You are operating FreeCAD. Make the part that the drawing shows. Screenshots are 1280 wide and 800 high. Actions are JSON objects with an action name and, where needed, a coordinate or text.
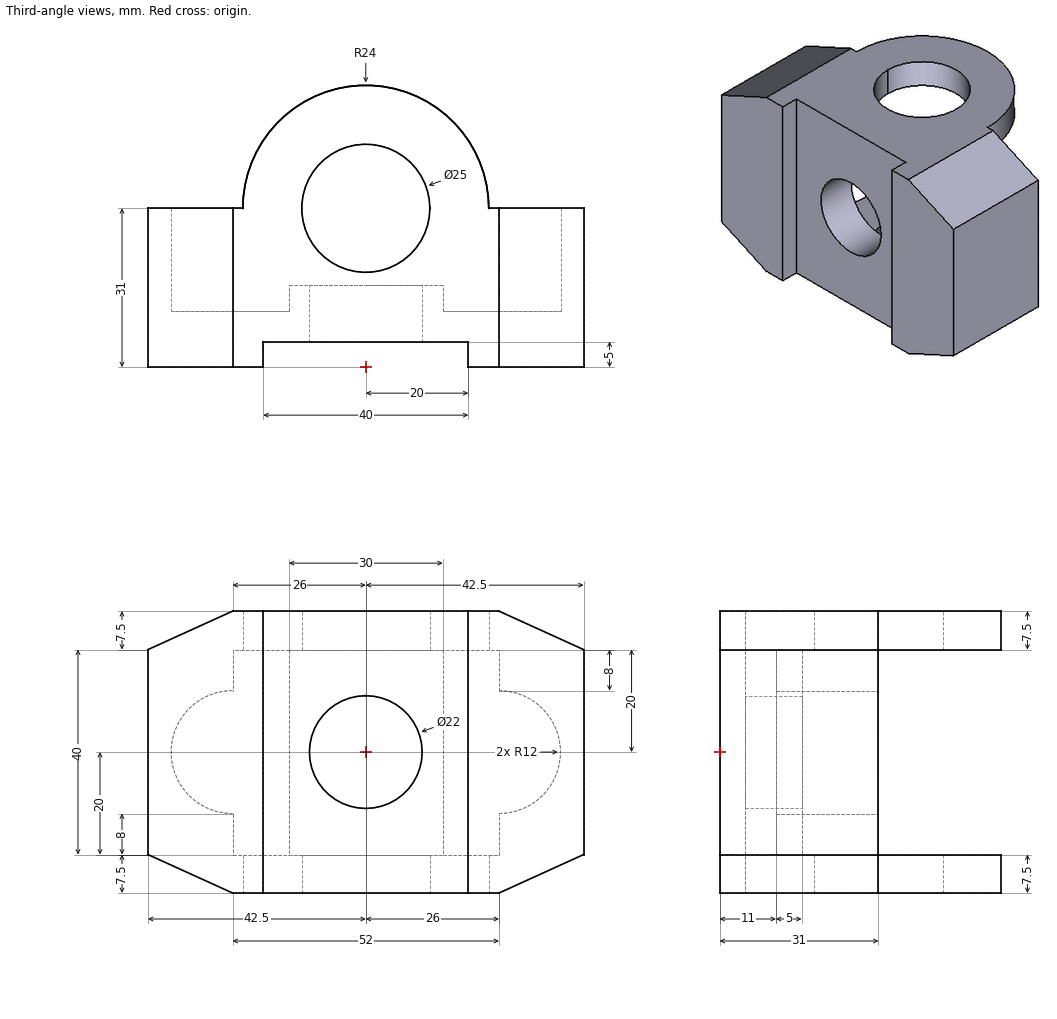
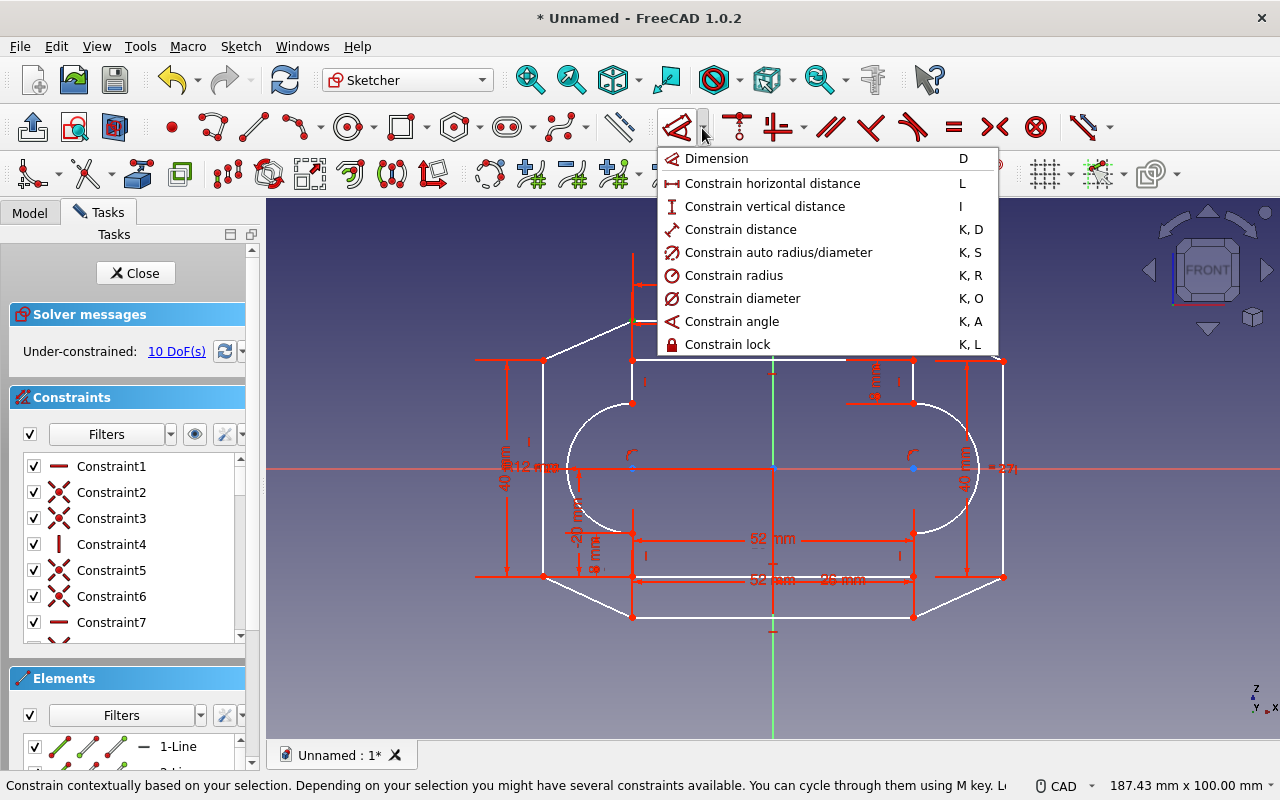
{"action": "left_click", "coordinate": [828, 184]}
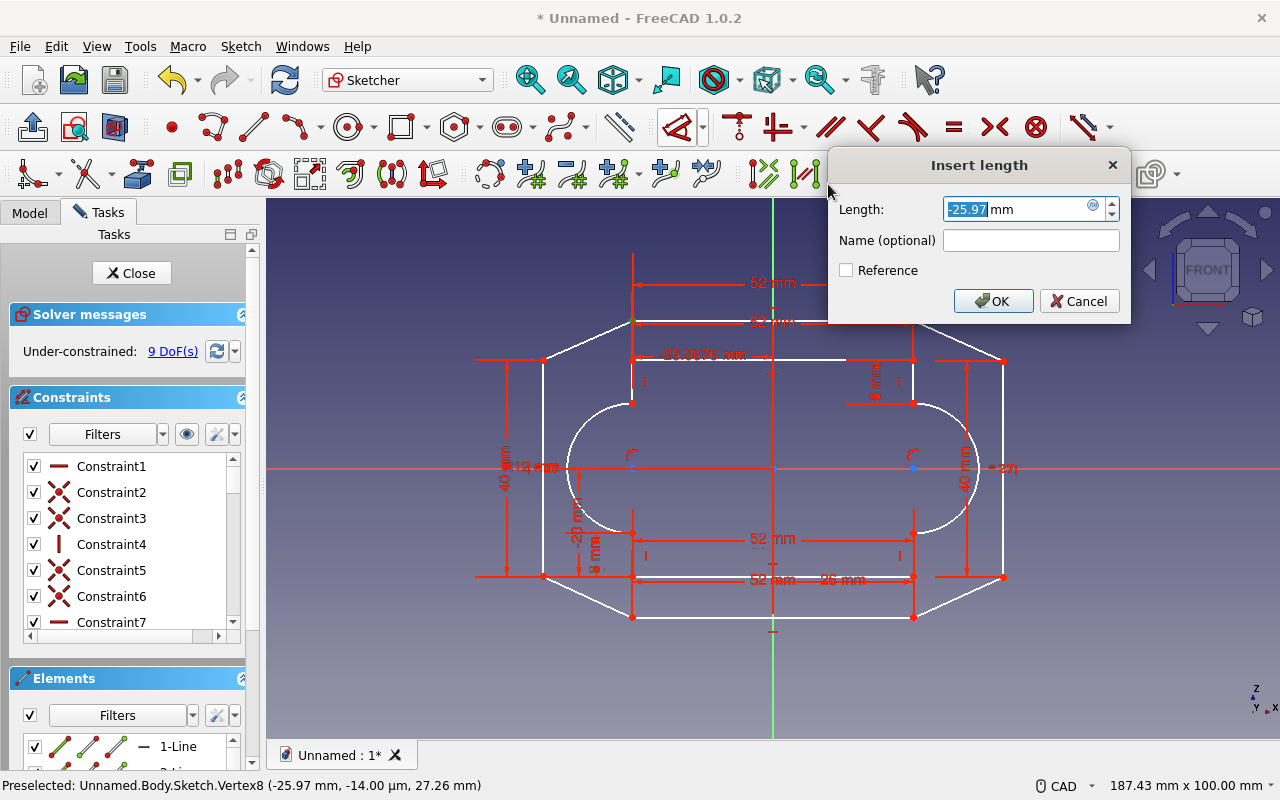
{"action": "type", "text": "-26"}
{"action": "key", "text": "Return"}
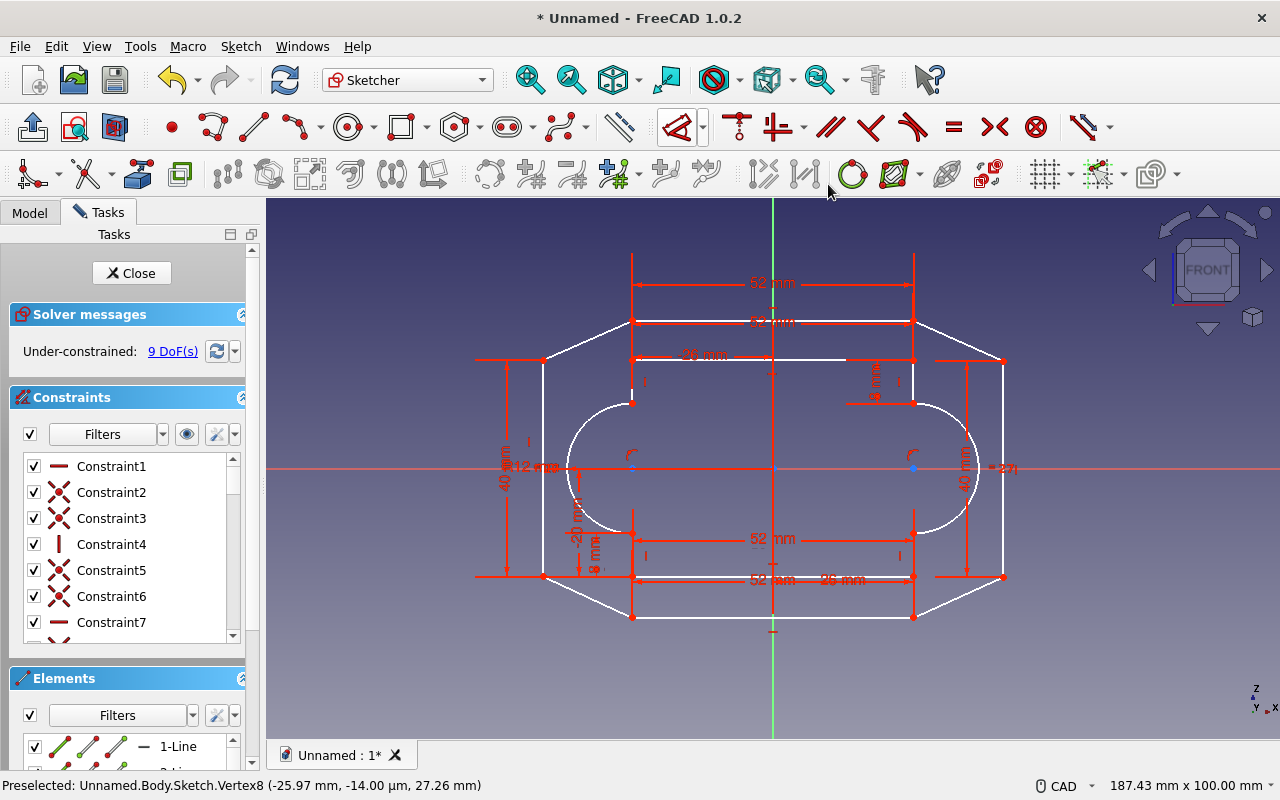
{"action": "left_click", "coordinate": [1003, 361]}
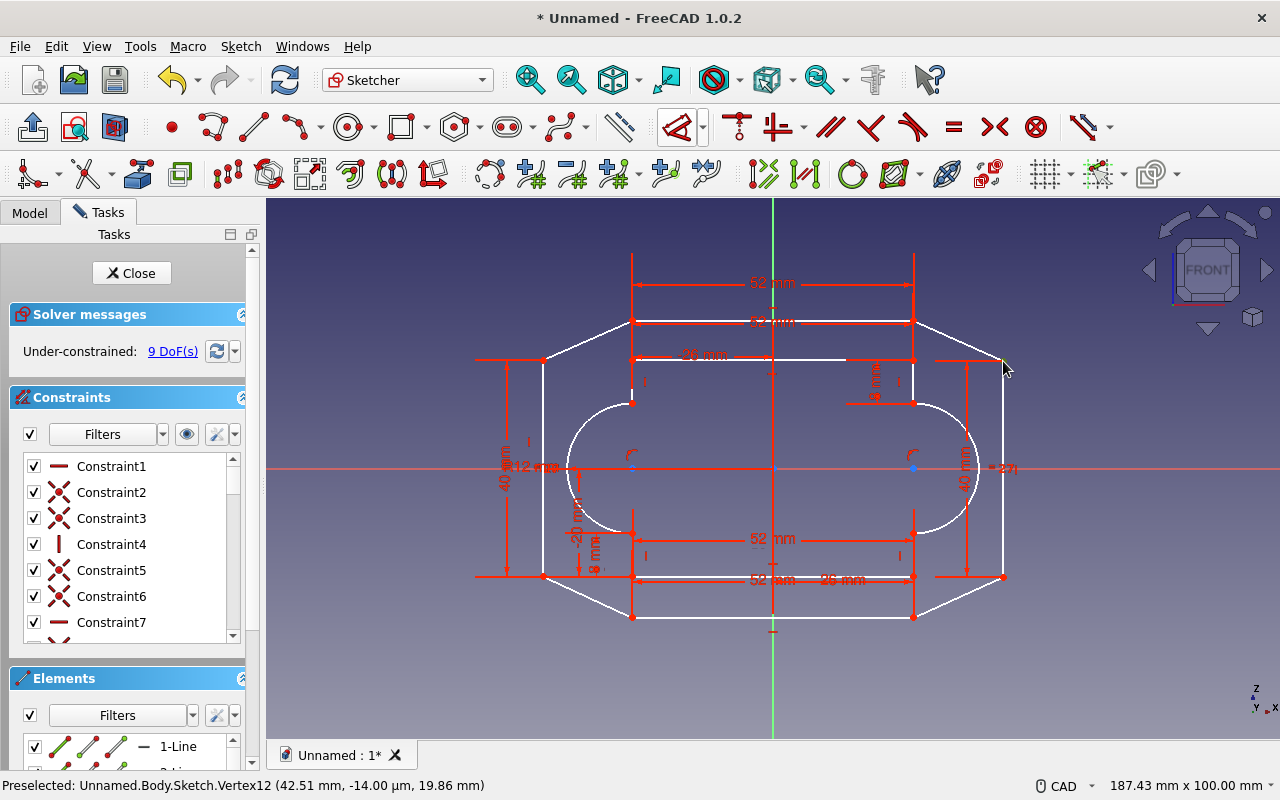
{"action": "left_click", "coordinate": [702, 128]}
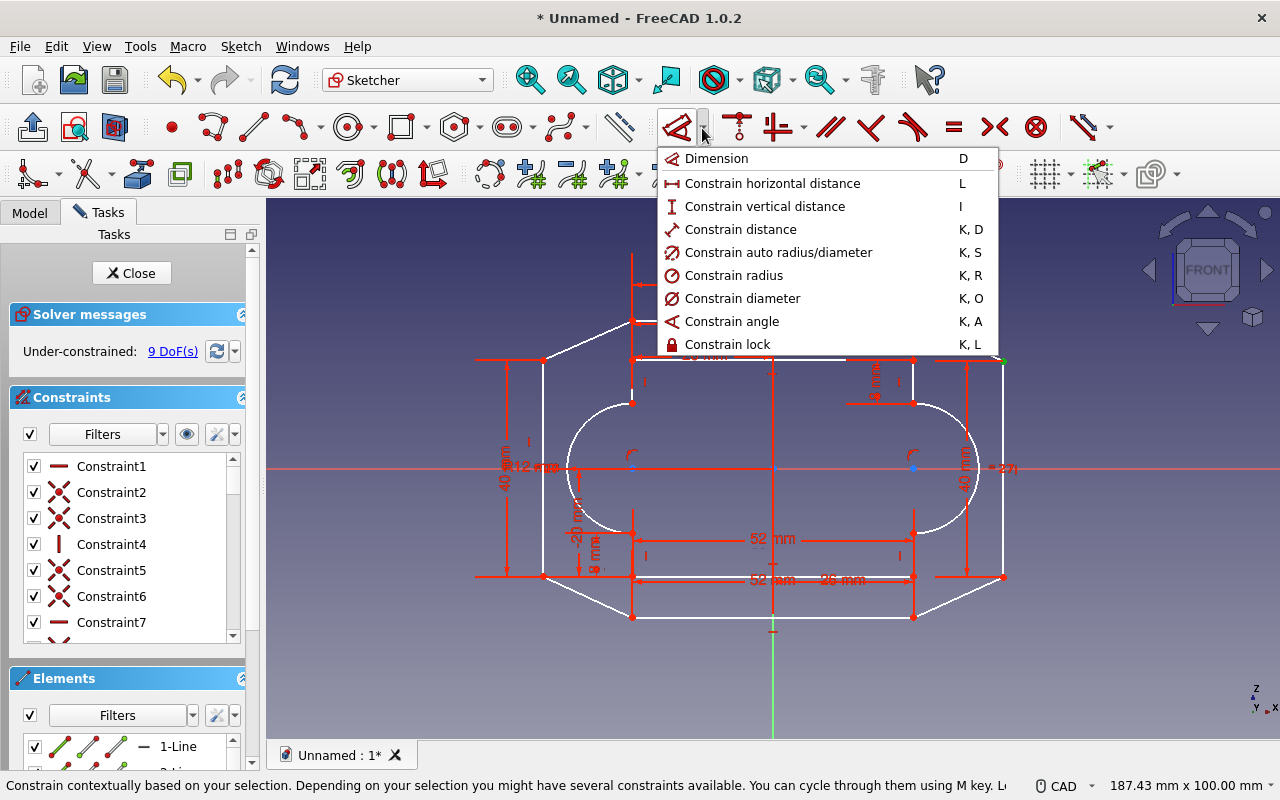
{"action": "left_click", "coordinate": [828, 206]}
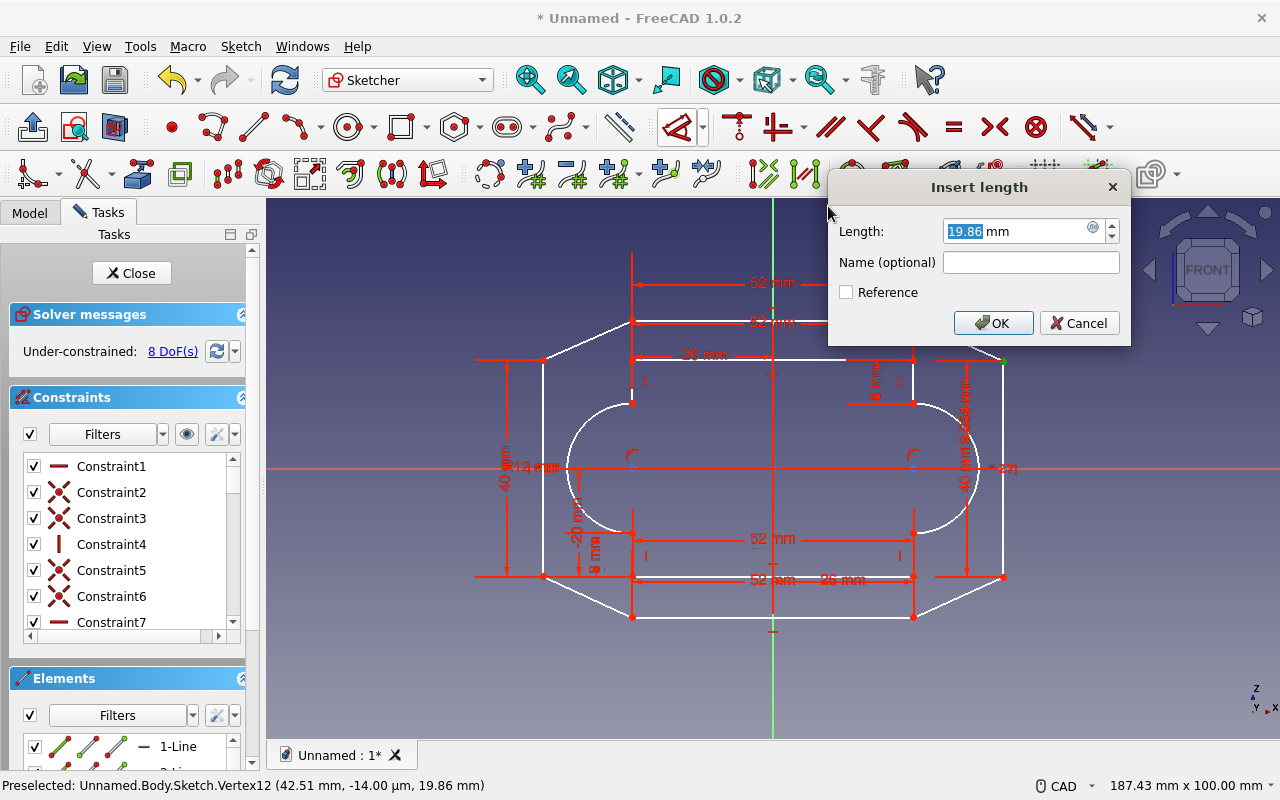
{"action": "type", "text": "20"}
{"action": "key", "text": "Return"}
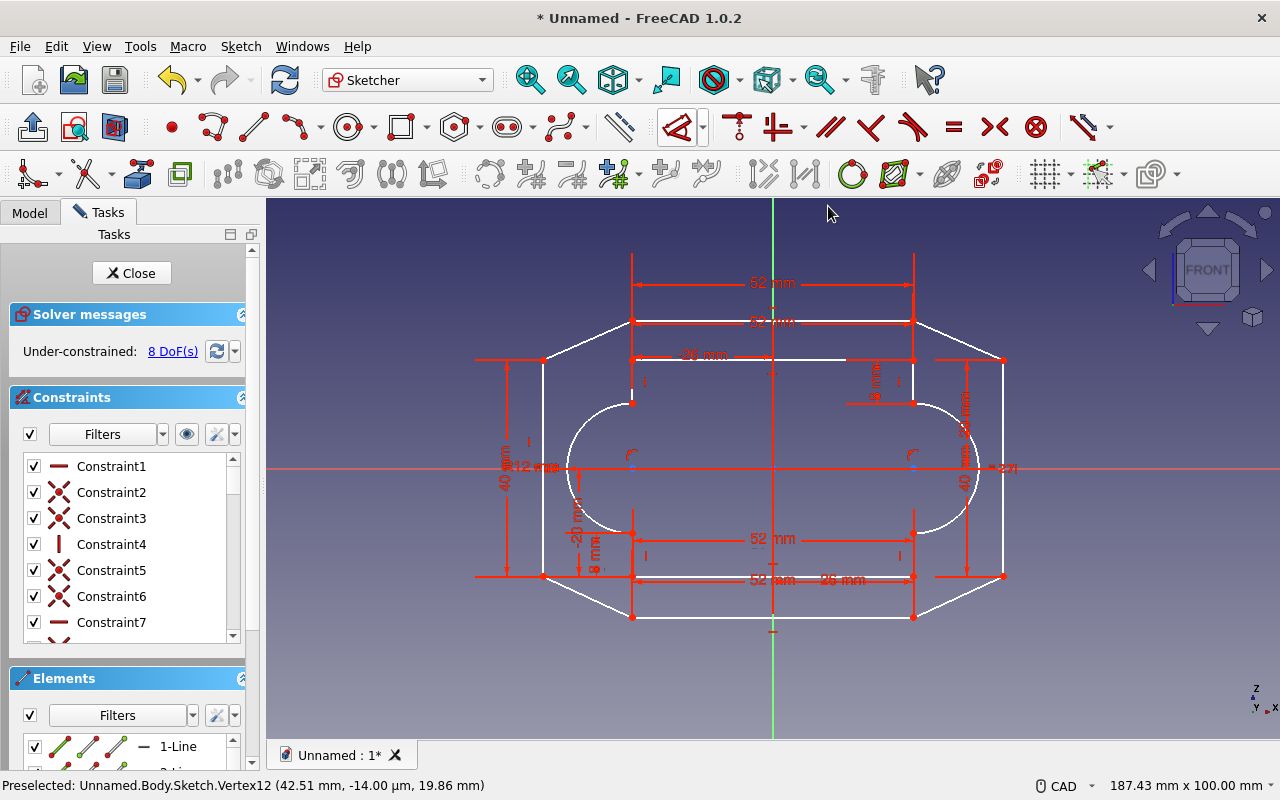
{"action": "left_click", "coordinate": [913, 404]}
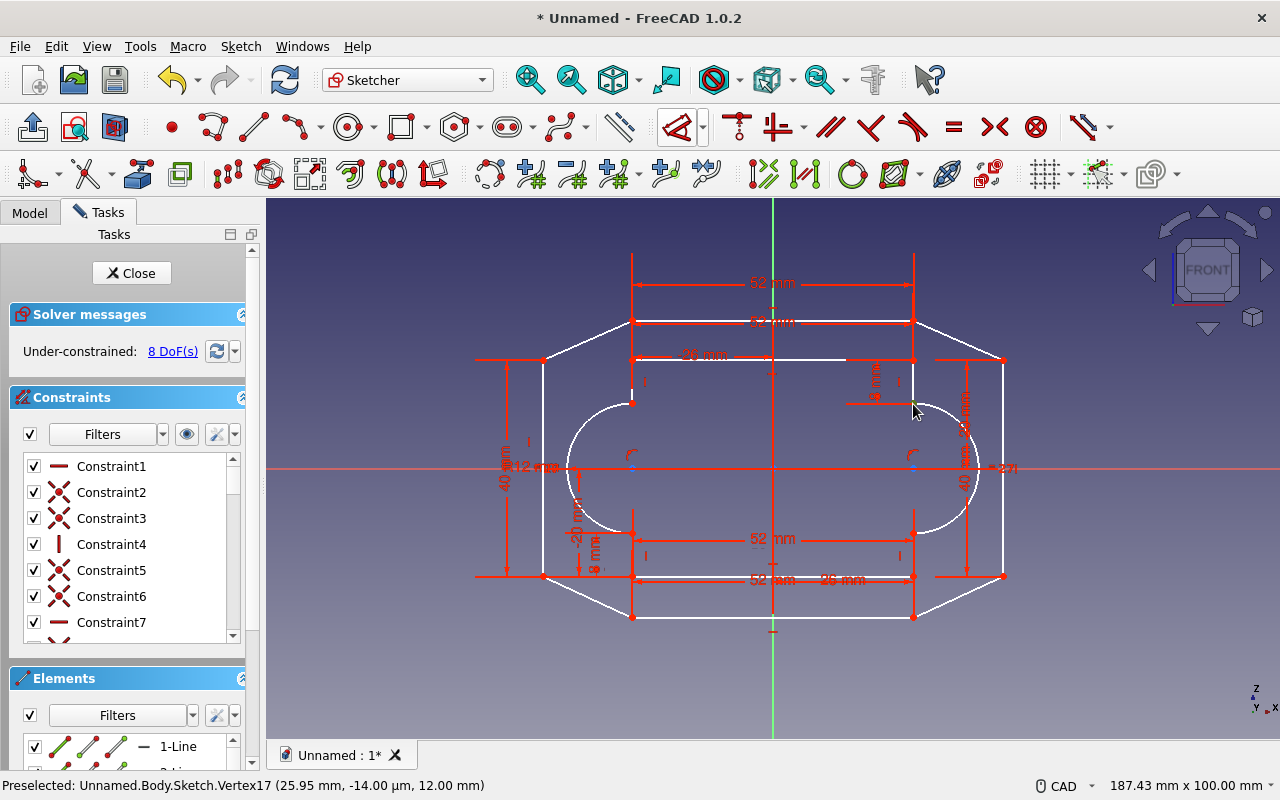
{"action": "key", "text": "l"}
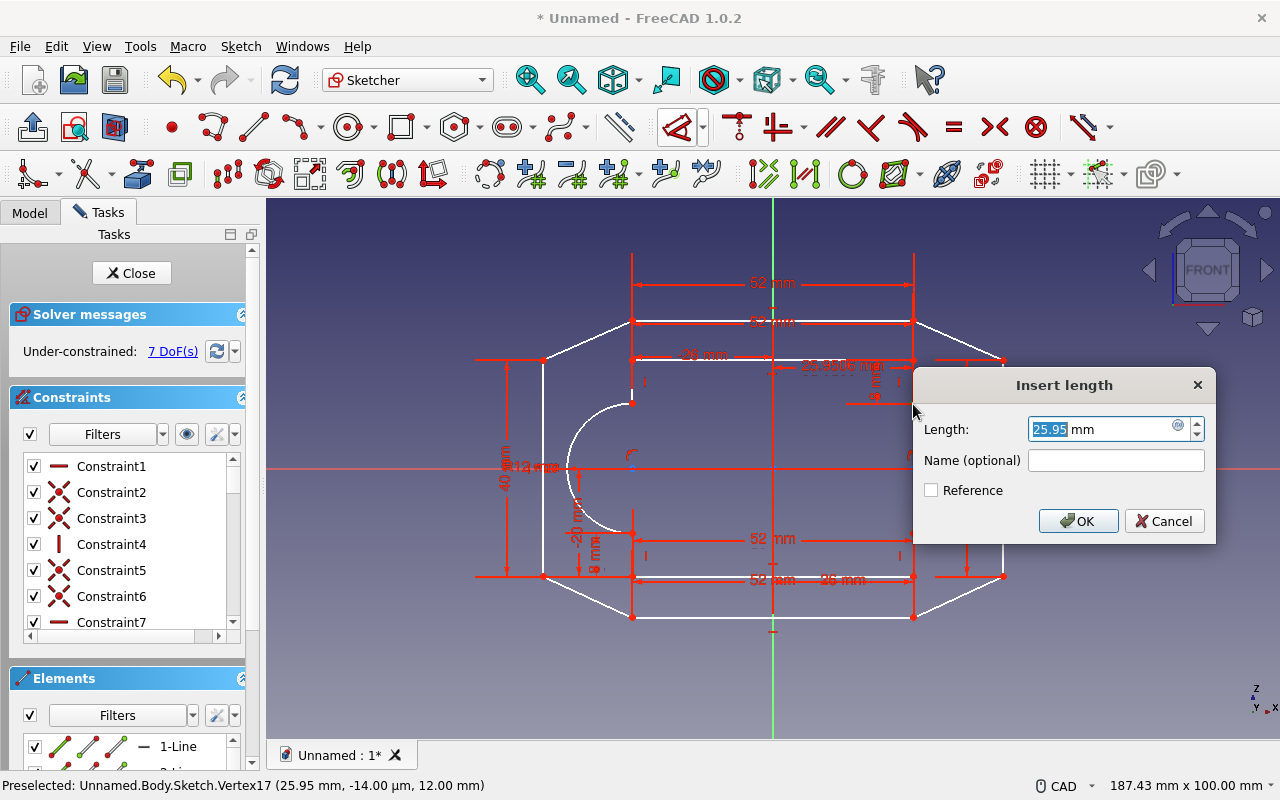
{"action": "type", "text": "26"}
{"action": "key", "text": "Return"}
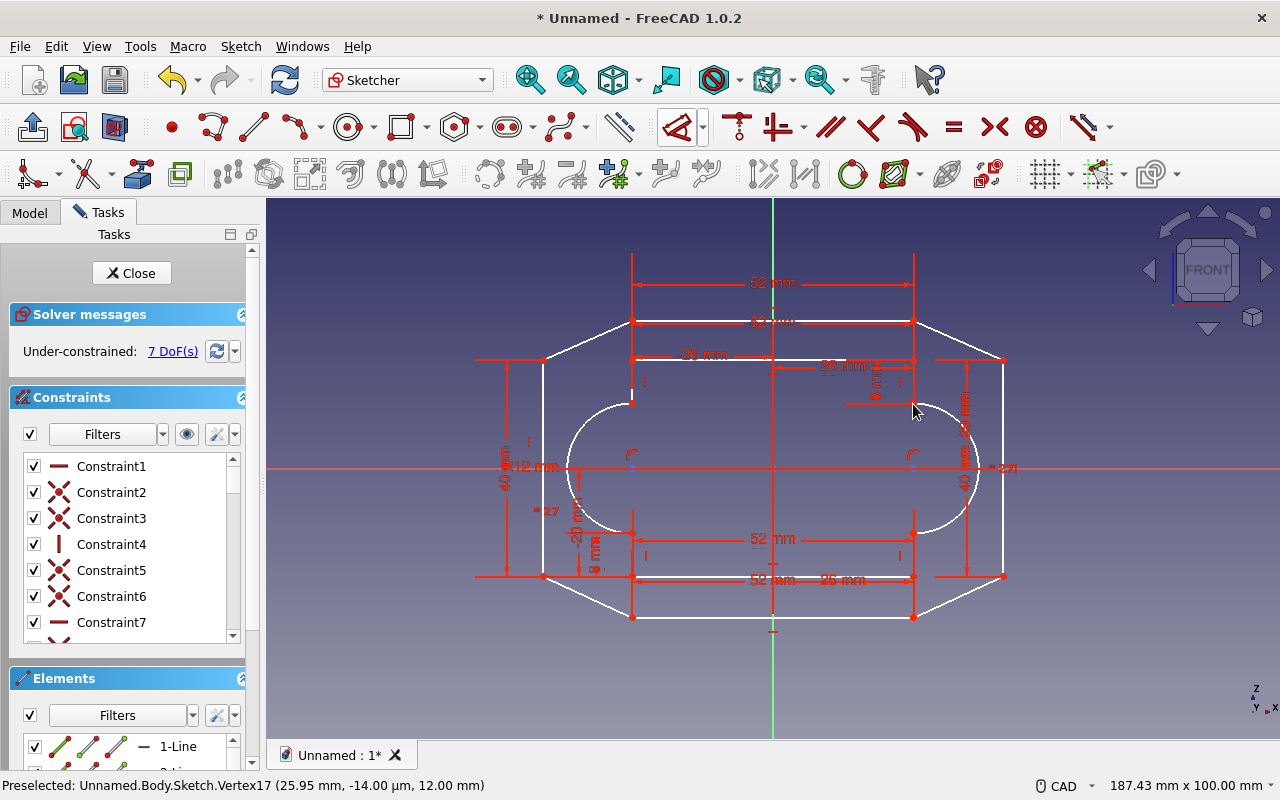
{"action": "left_click", "coordinate": [633, 533]}